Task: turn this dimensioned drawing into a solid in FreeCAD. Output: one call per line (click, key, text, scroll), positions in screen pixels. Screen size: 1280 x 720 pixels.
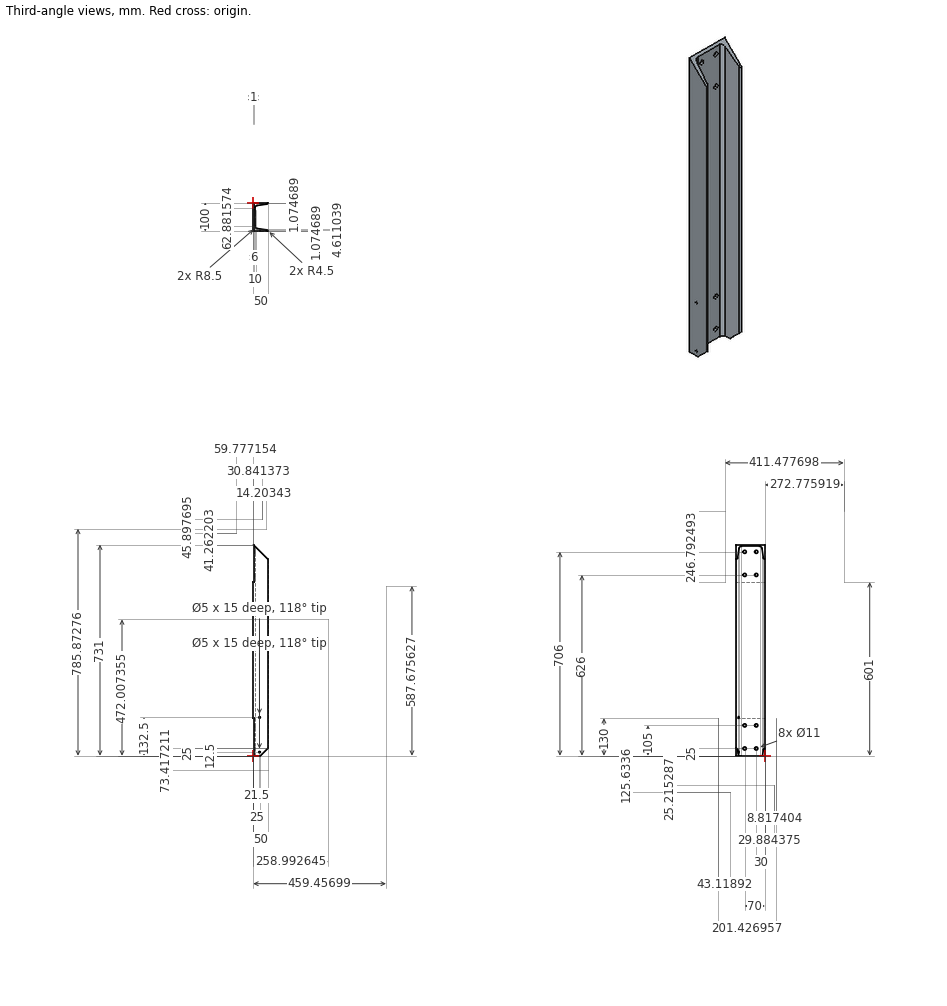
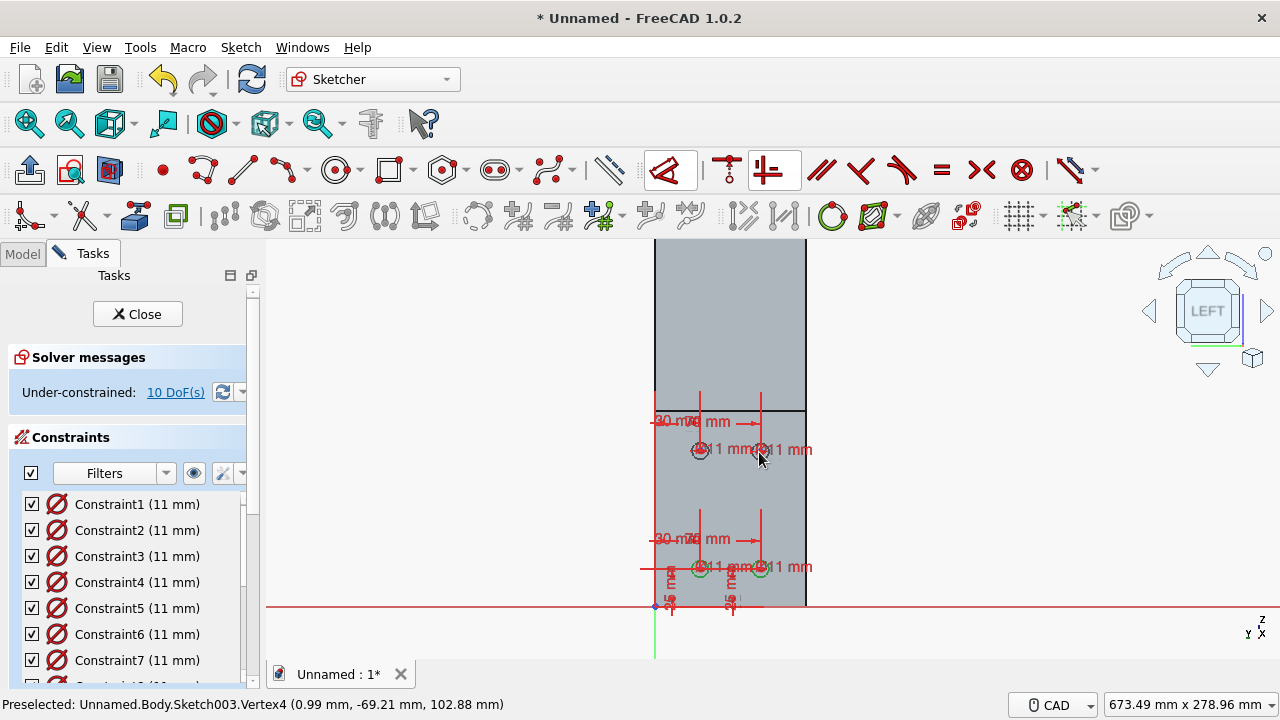
scroll(702, 573, down, 7)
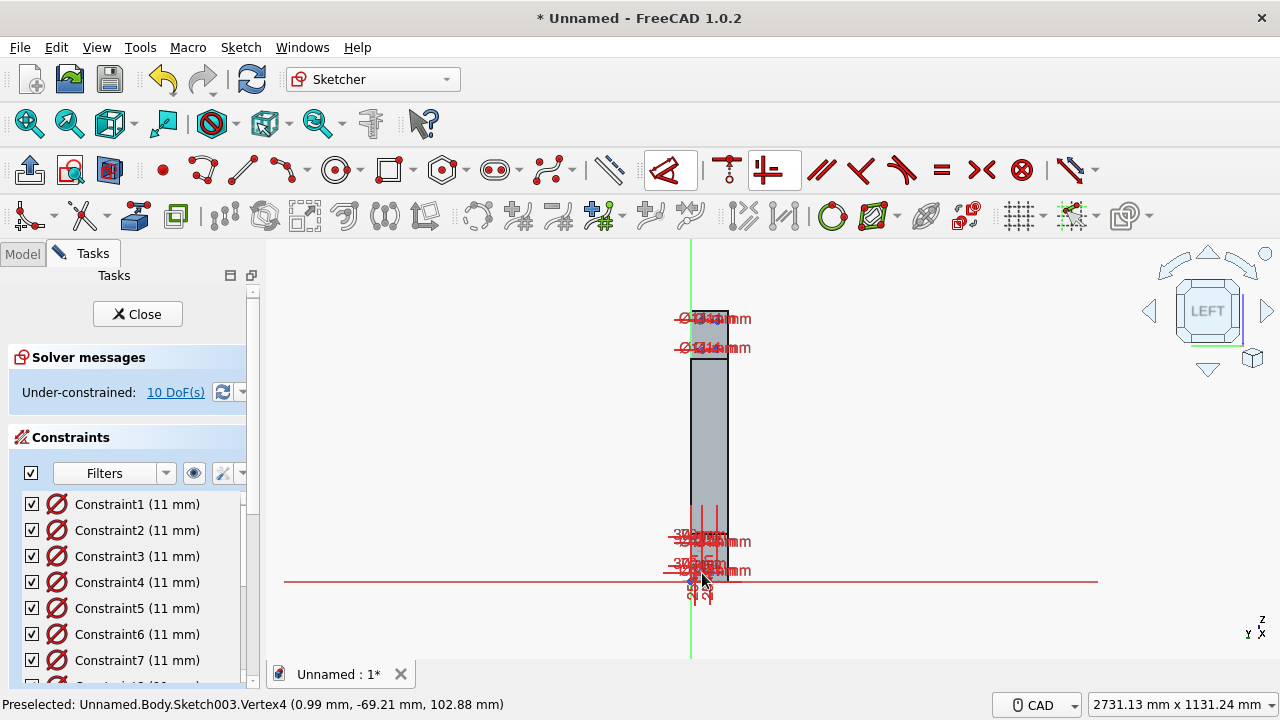
scroll(702, 350, up, 7)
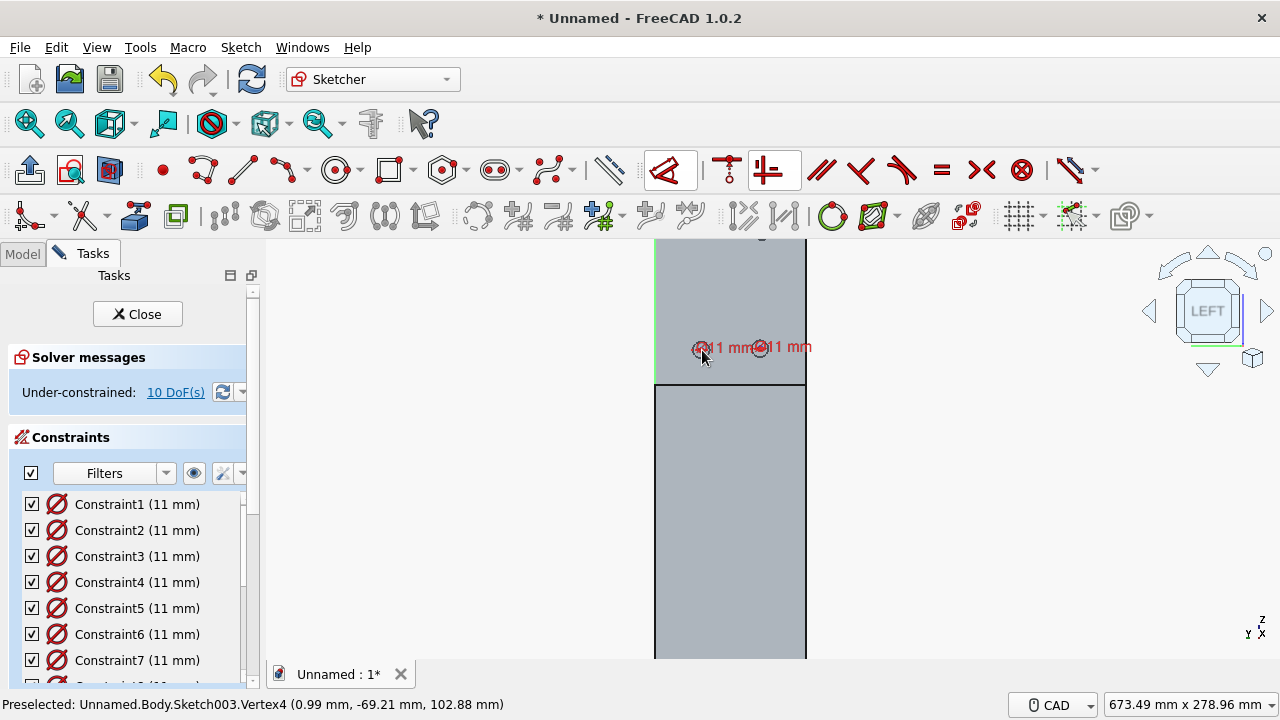
click(701, 350)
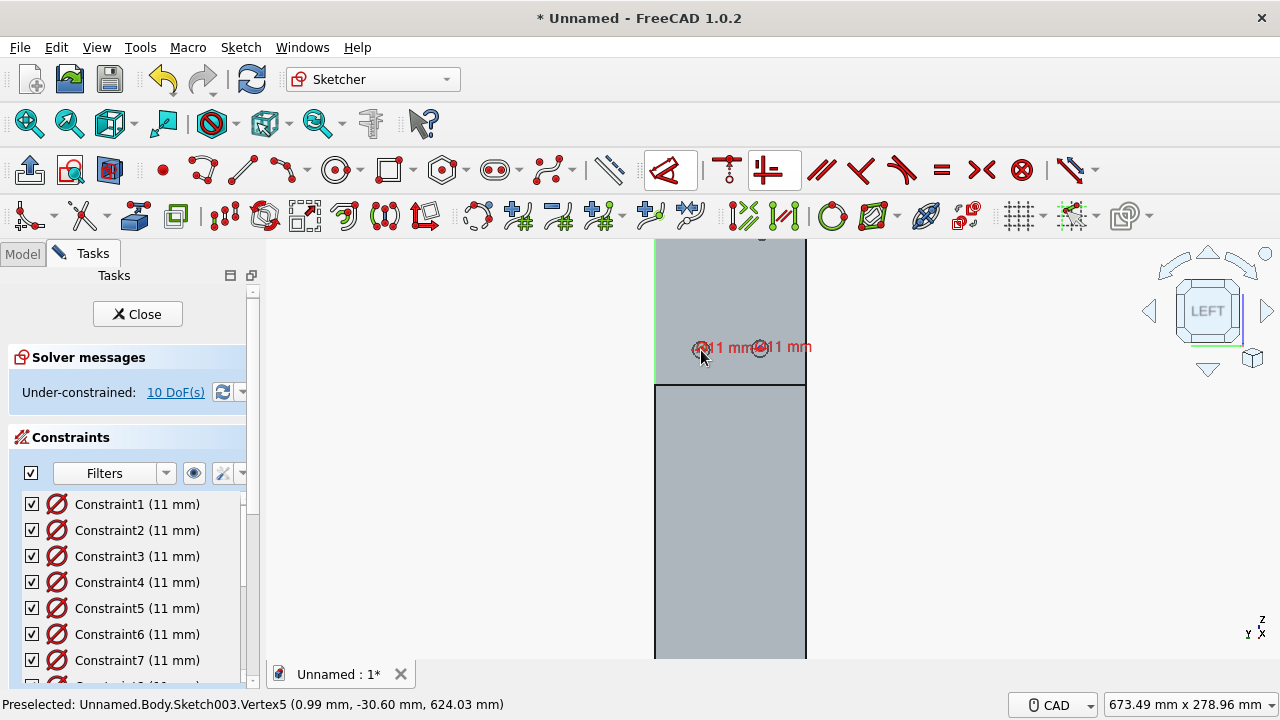
key(l)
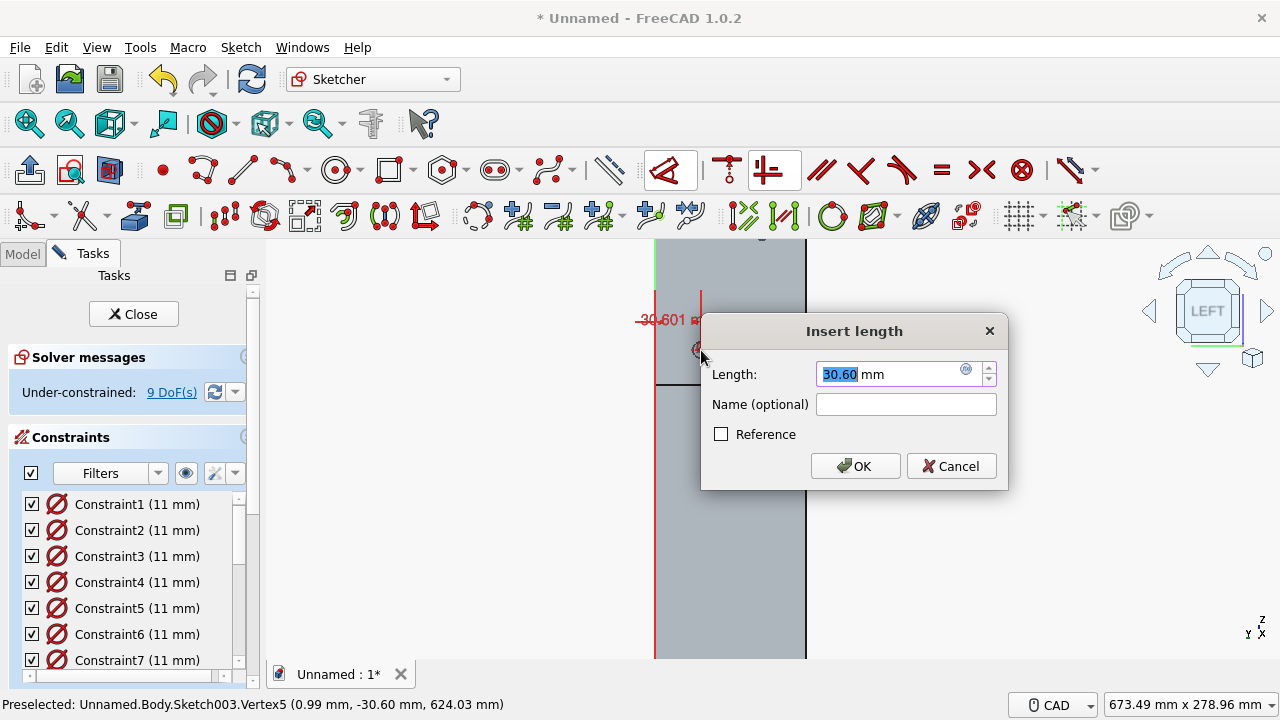
text(30)
key(Return)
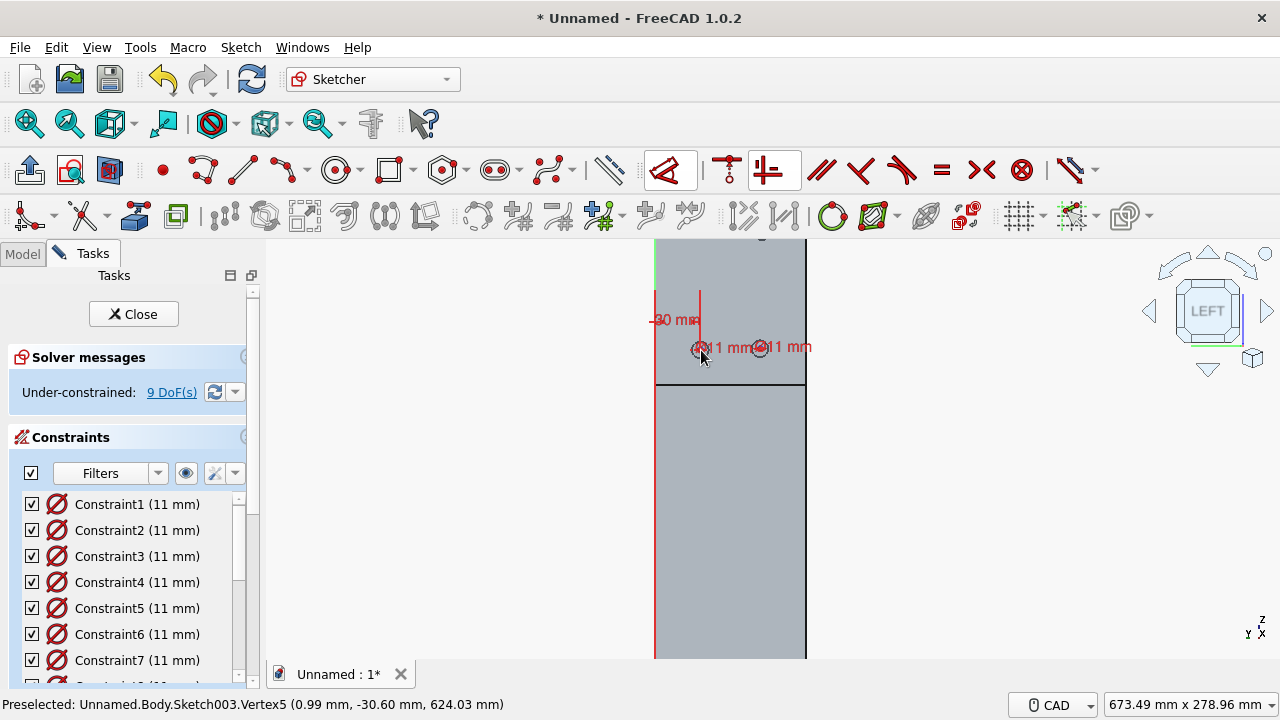
scroll(702, 349, down, 7)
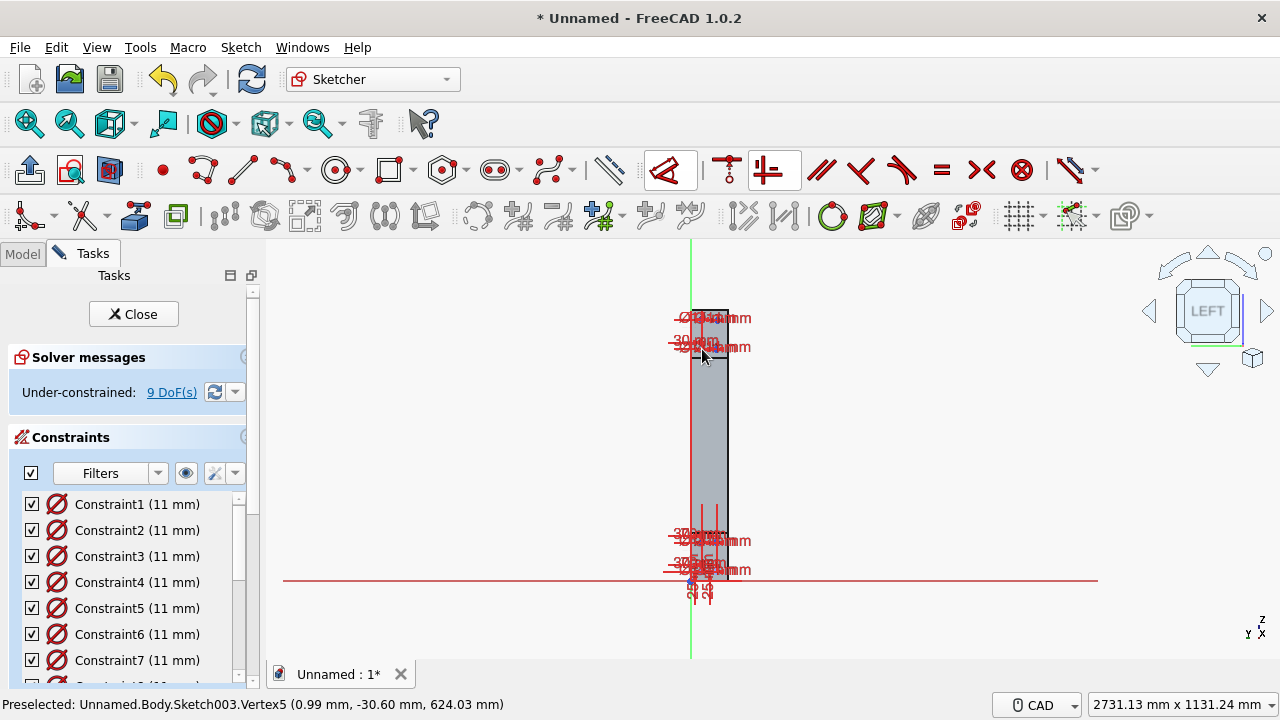
scroll(717, 320, up, 3)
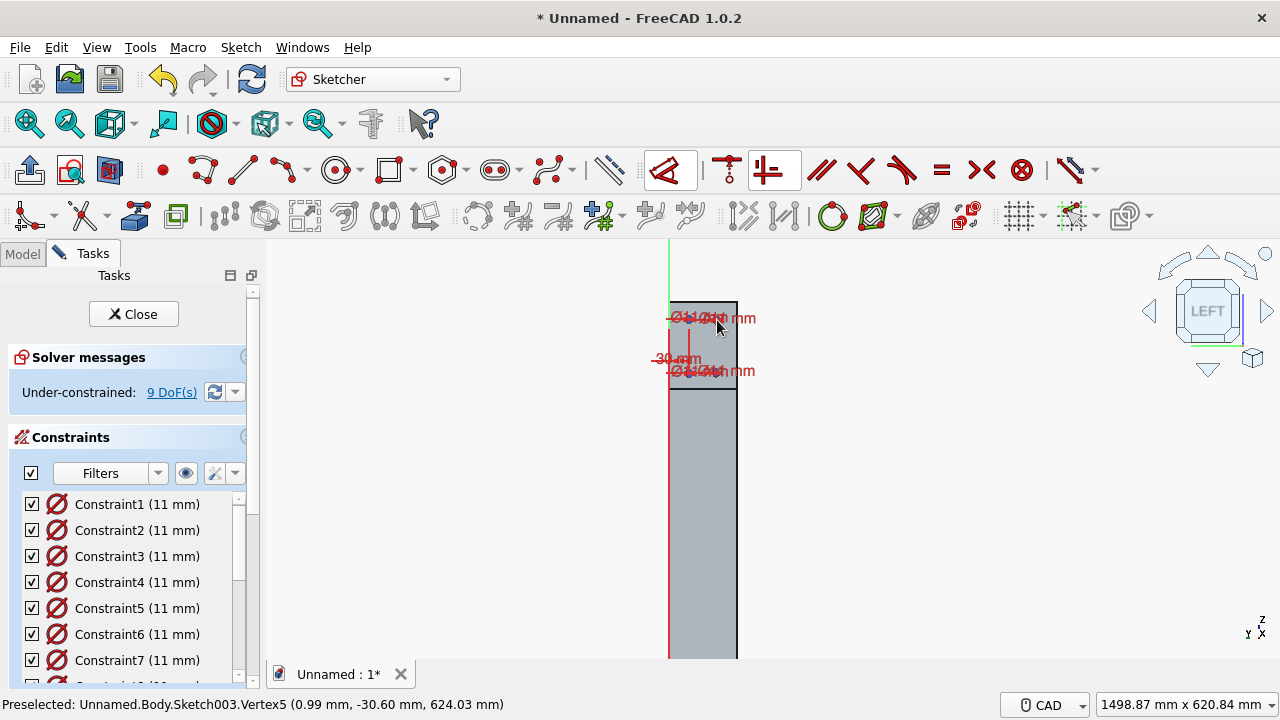
click(717, 320)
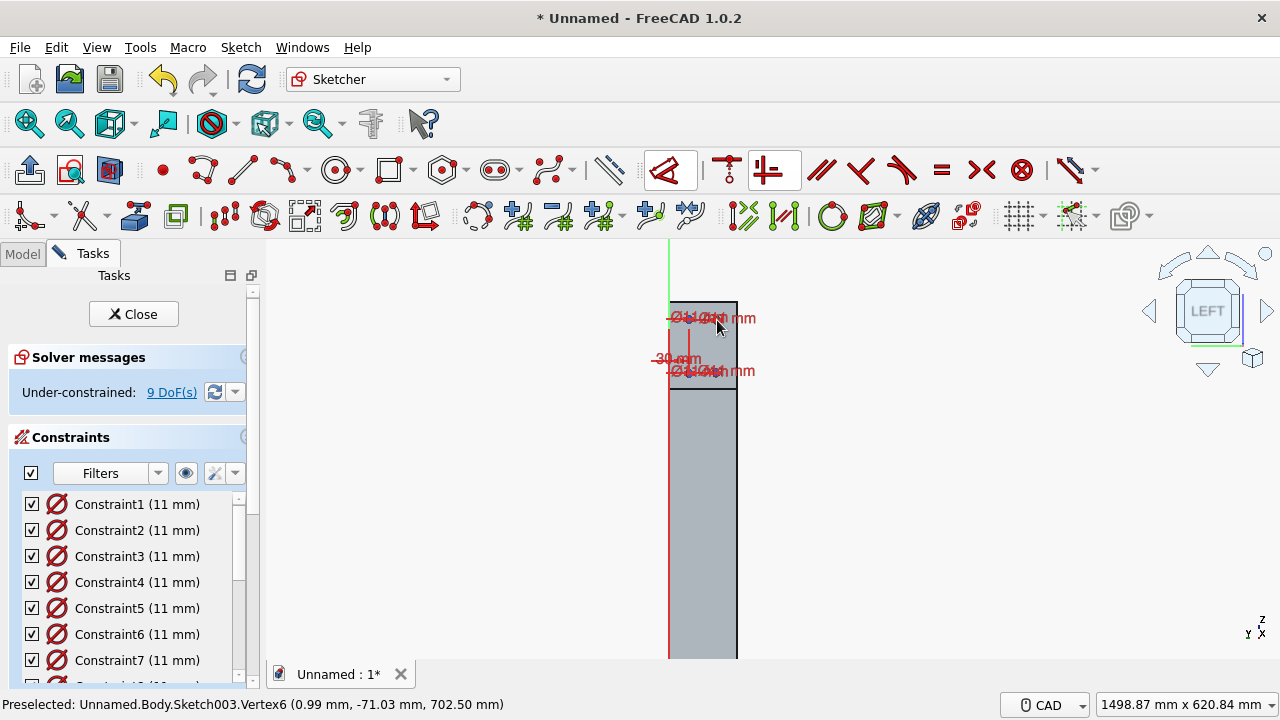
key(l)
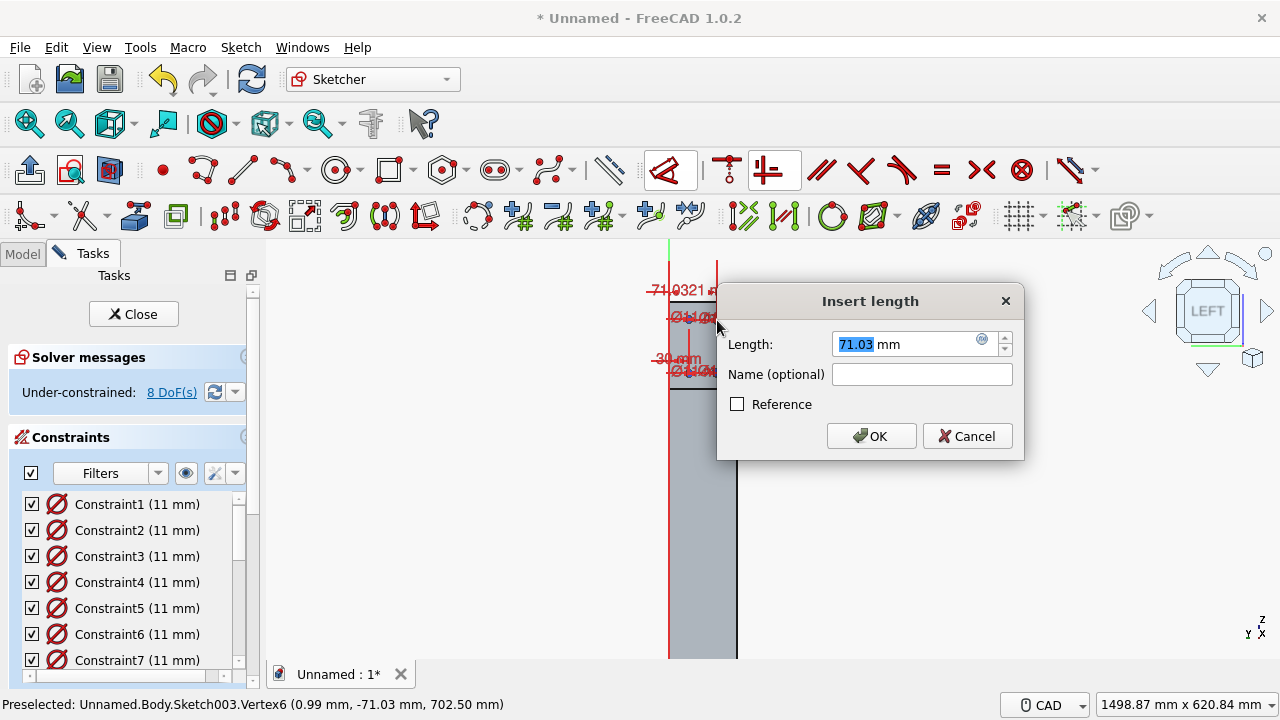
text(70)
key(Return)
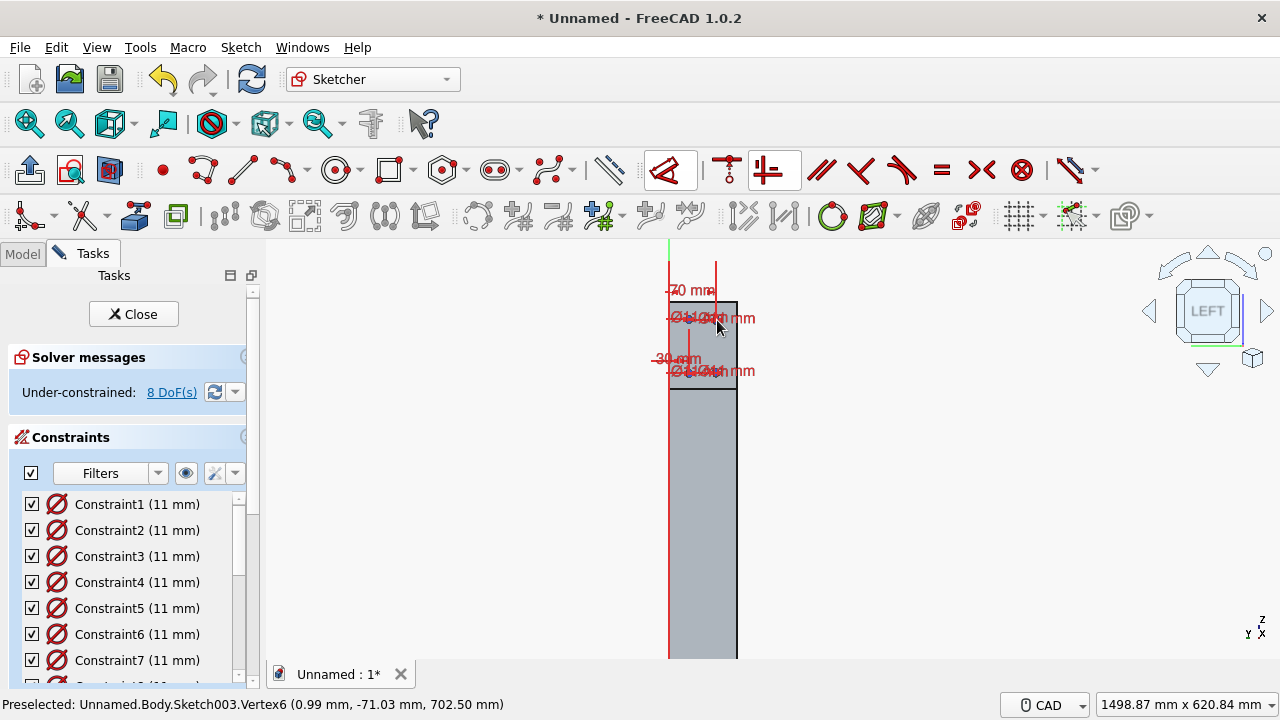
click(716, 373)